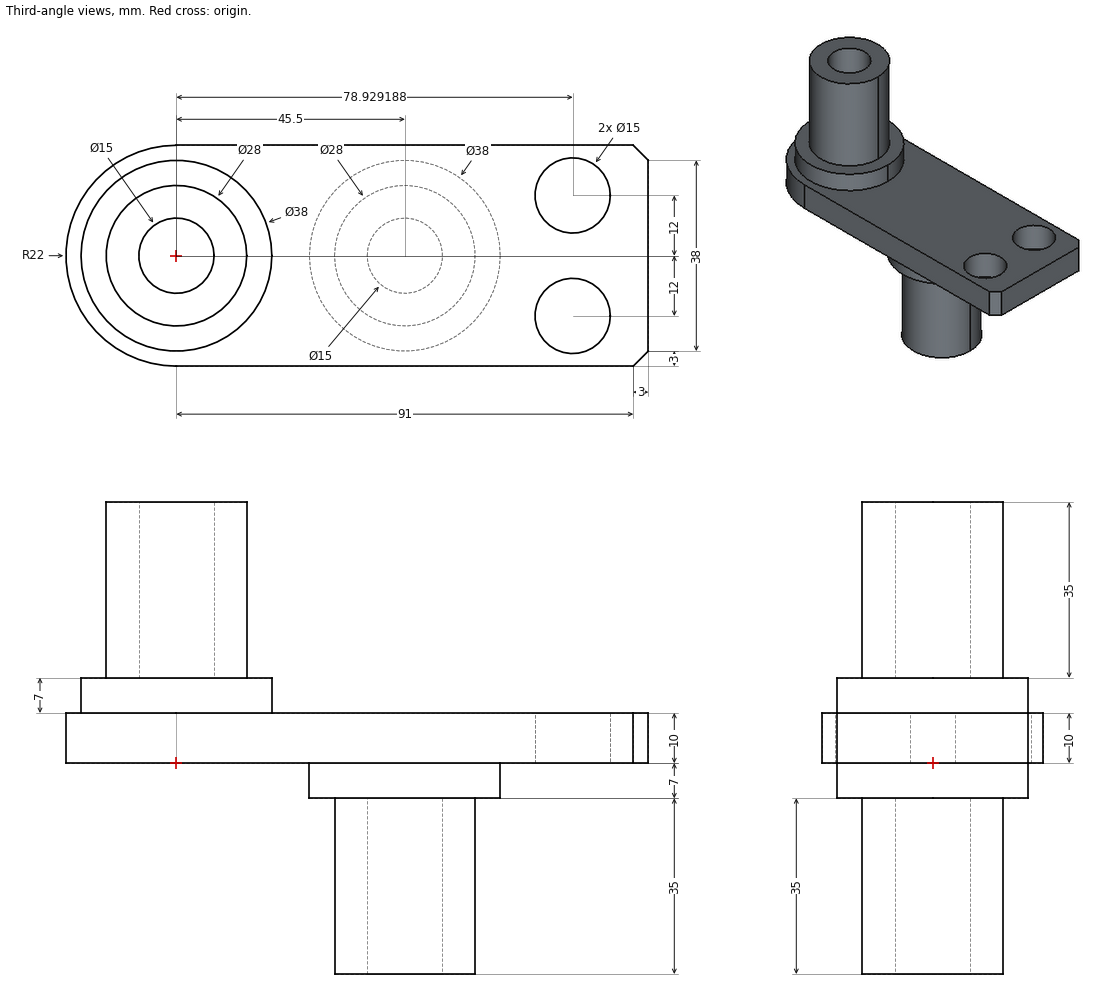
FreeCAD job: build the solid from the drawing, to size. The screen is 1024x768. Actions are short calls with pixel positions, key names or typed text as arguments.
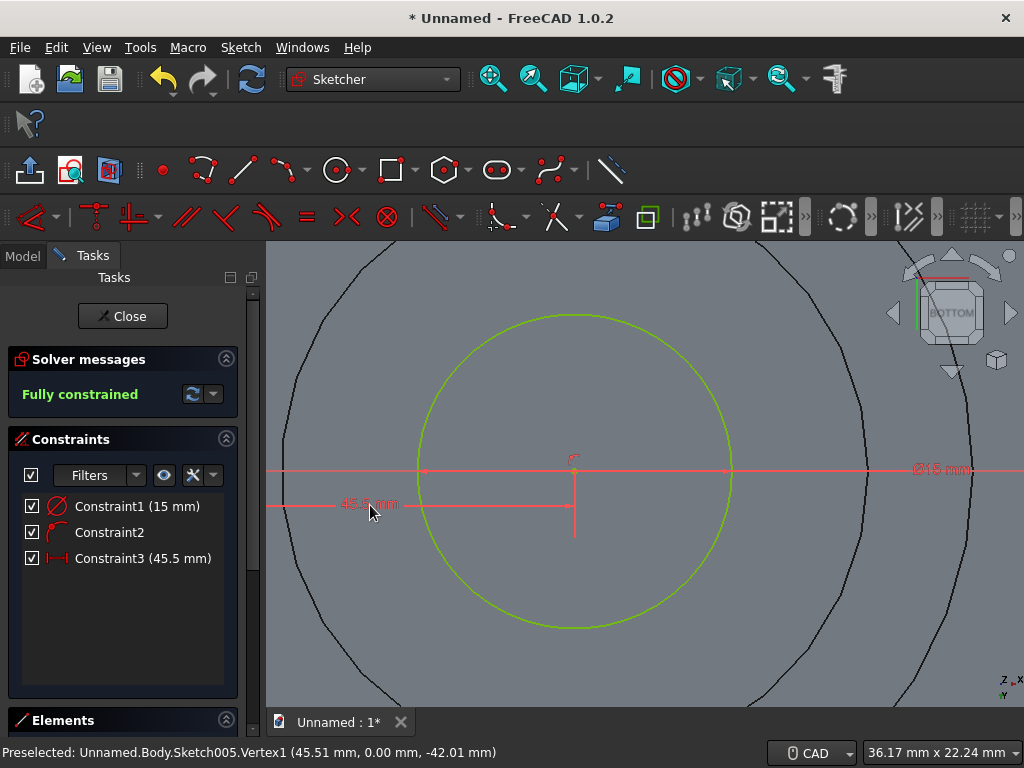
click(123, 316)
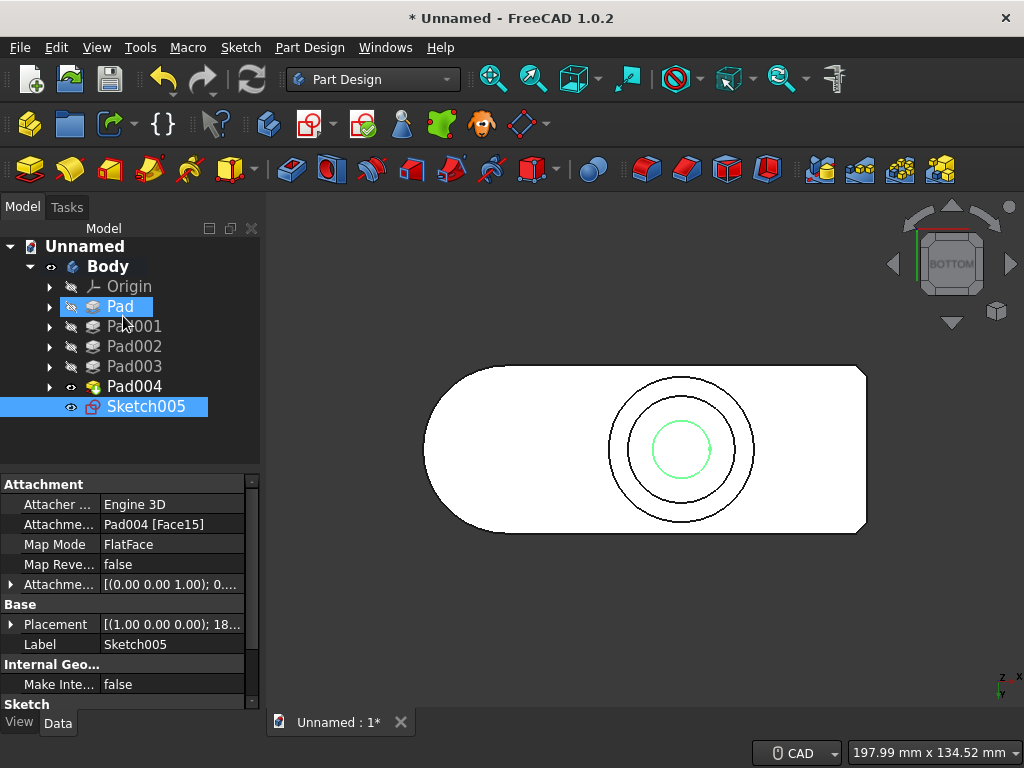
click(292, 170)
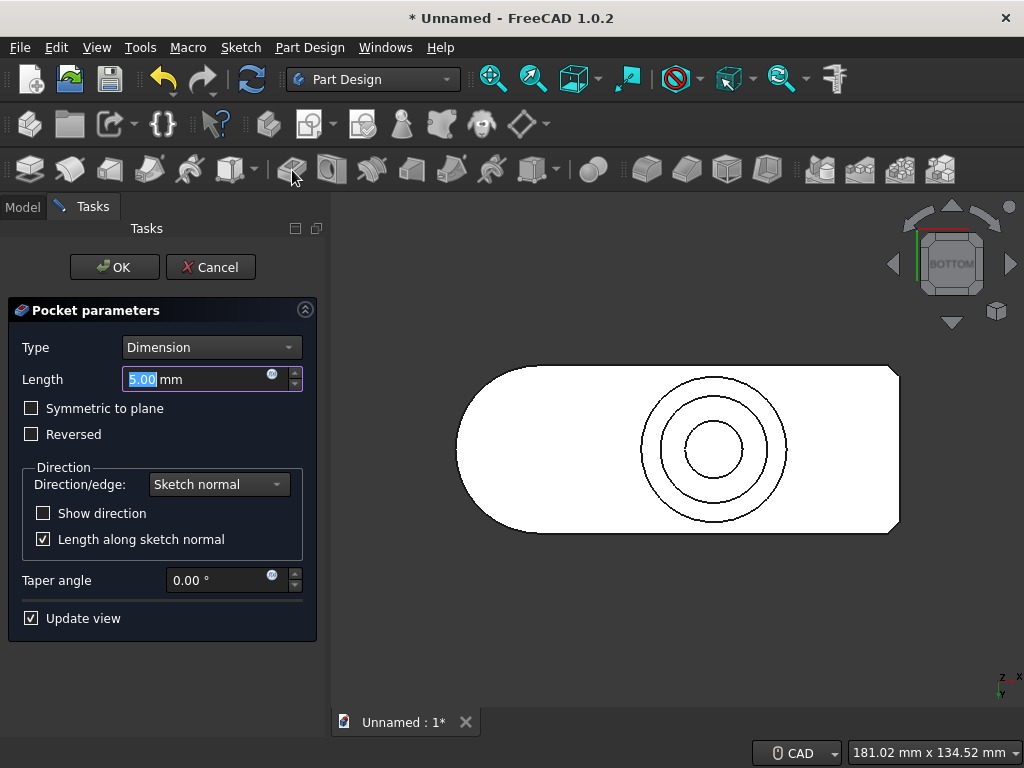
text(35)
key(Tab)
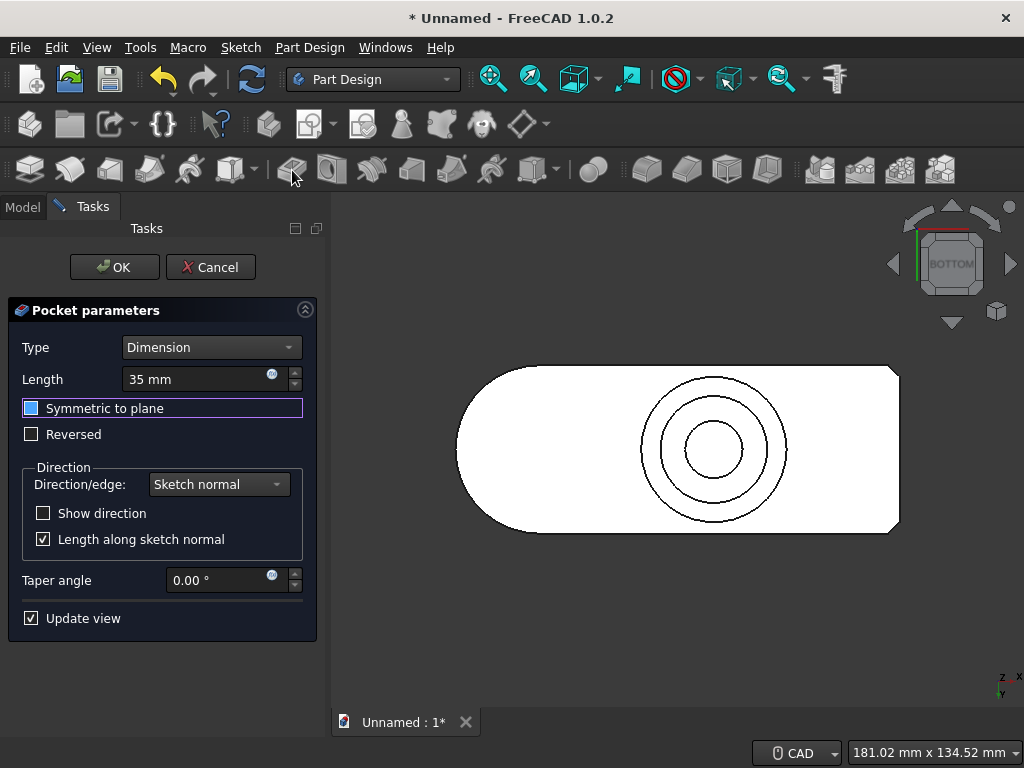
click(115, 267)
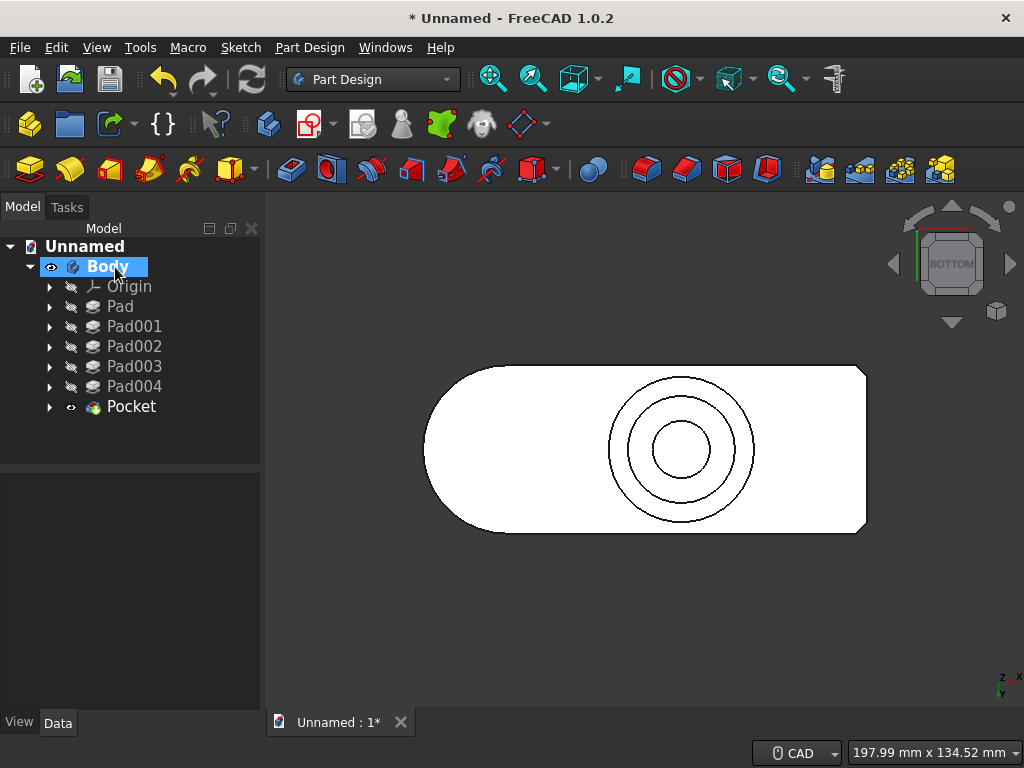
key(0)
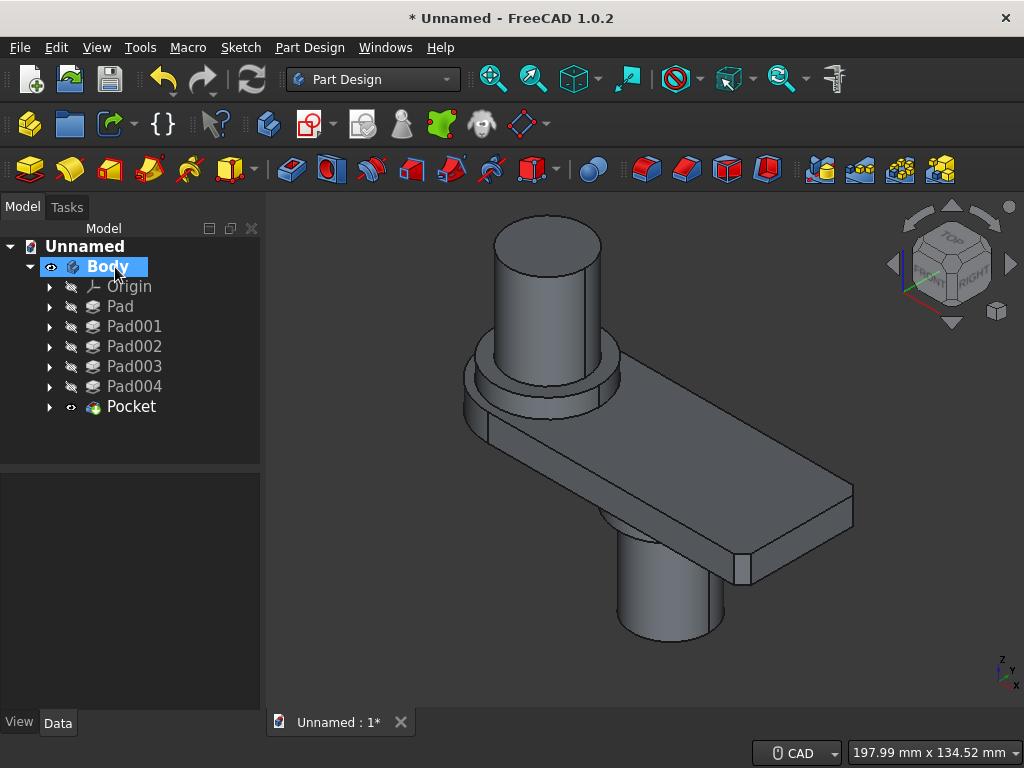
click(494, 80)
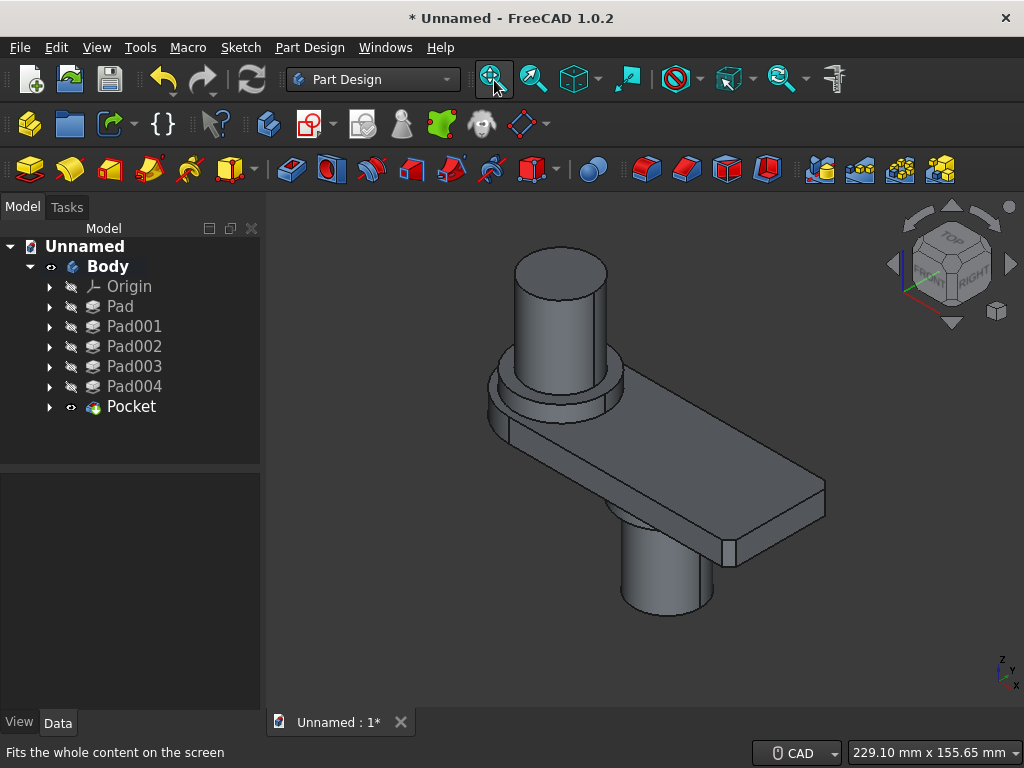
click(561, 273)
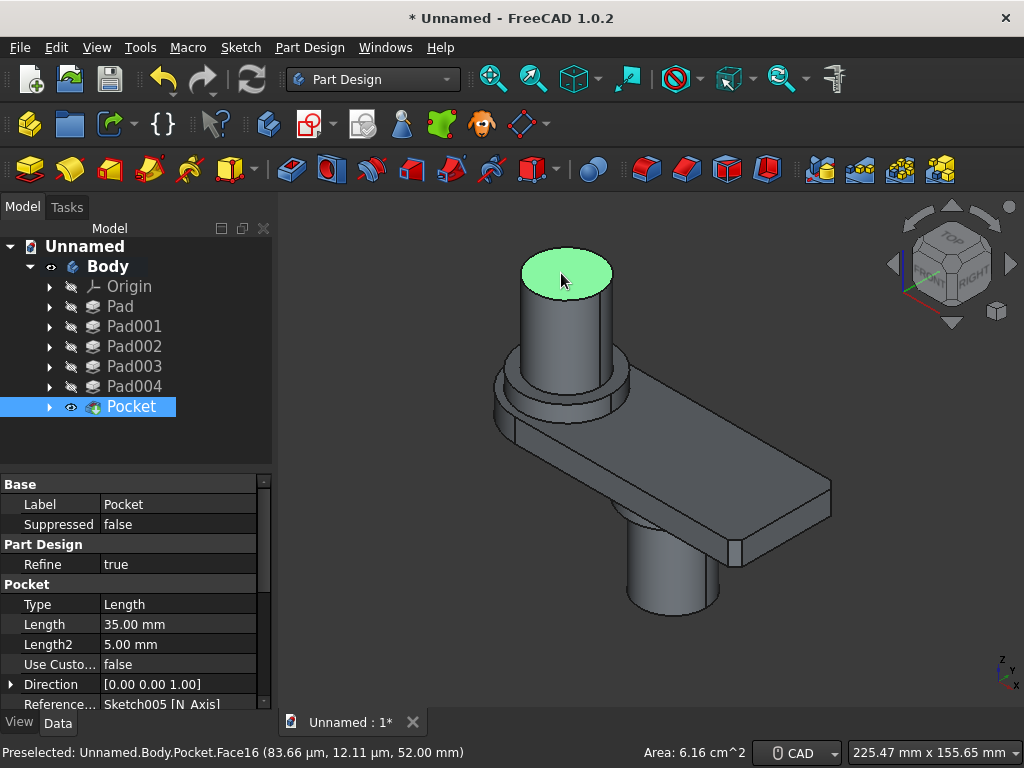
click(310, 124)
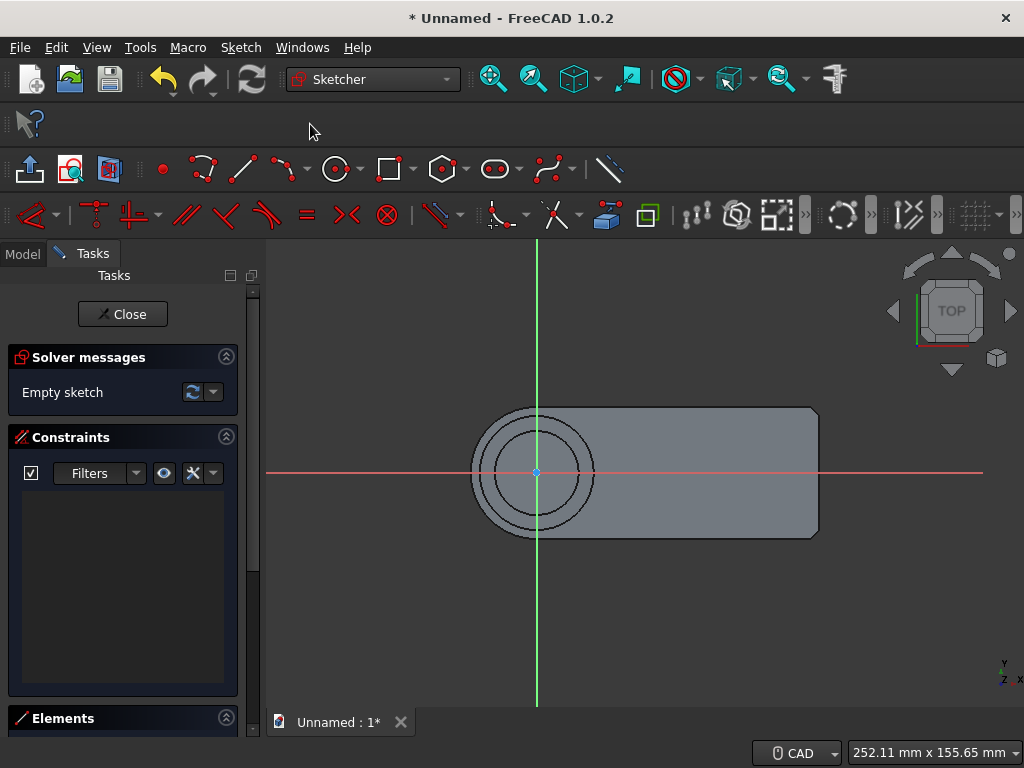
scroll(529, 473, up, 9)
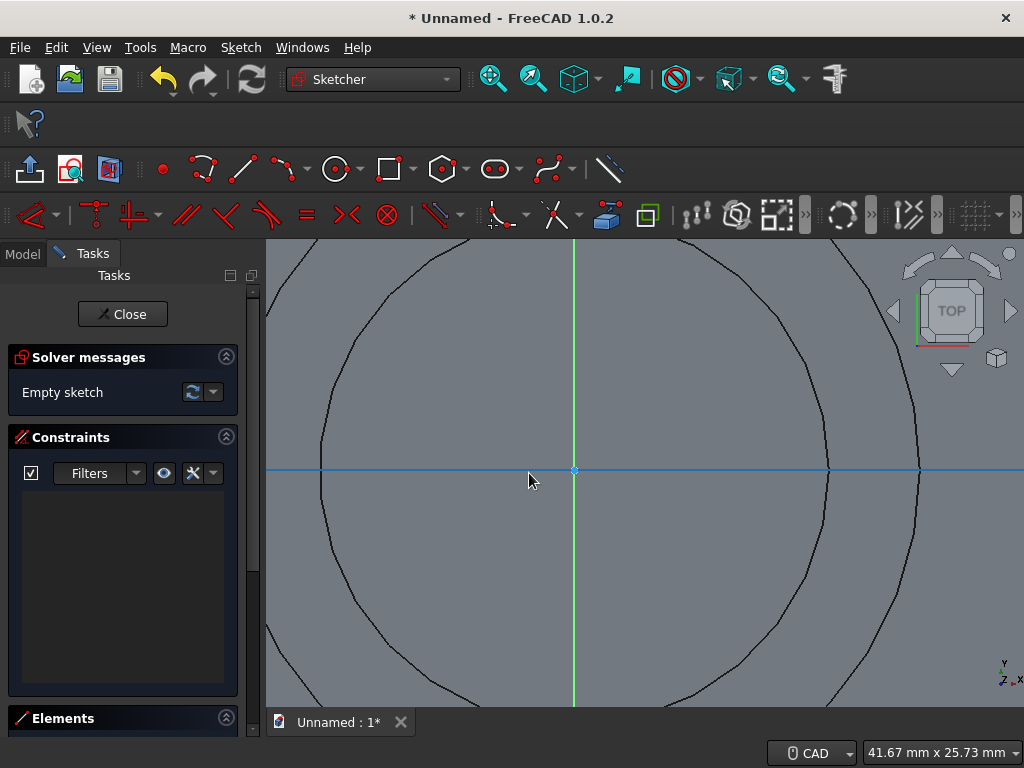
click(336, 170)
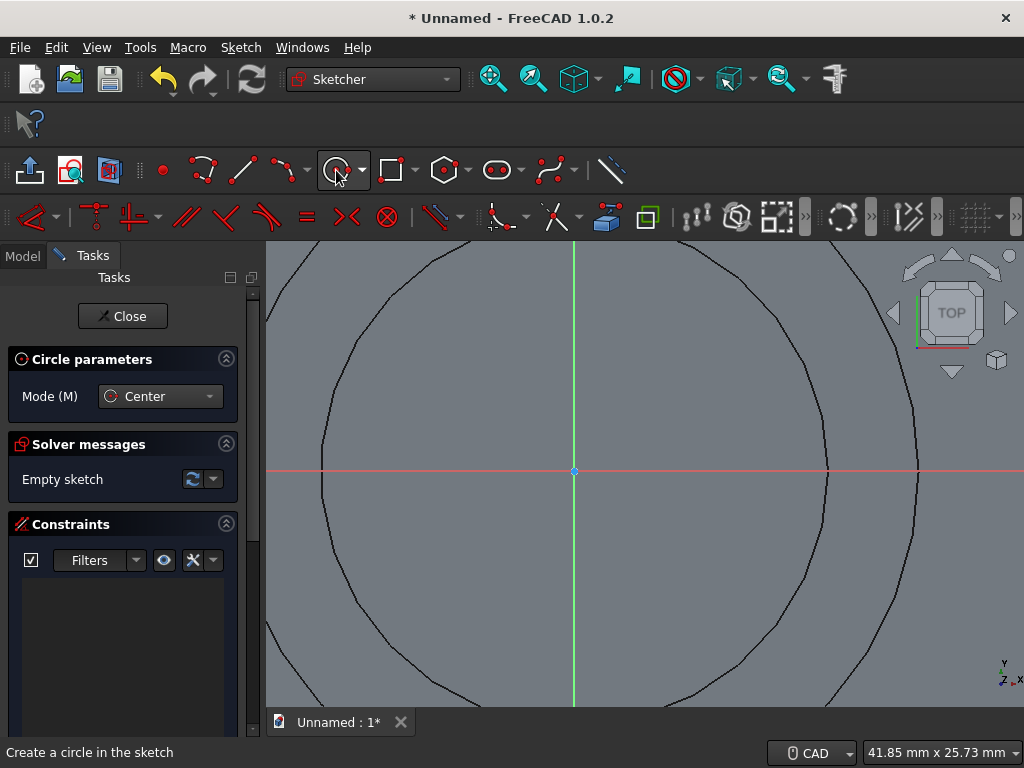
click(574, 471)
move(671, 375)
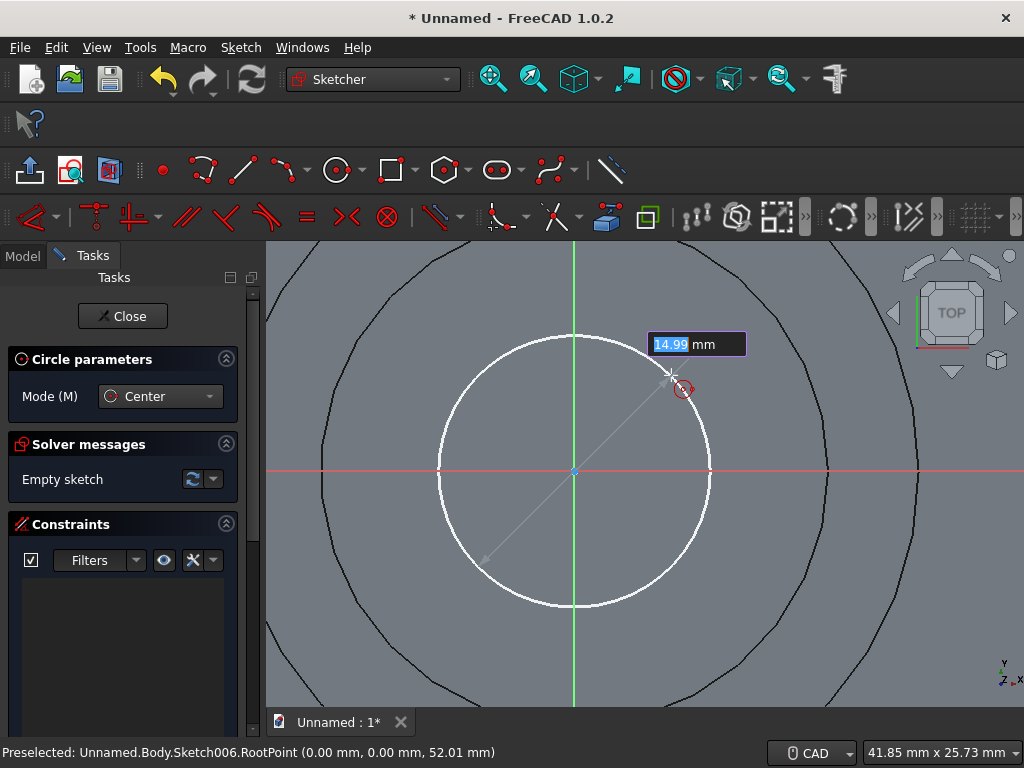
text(15)
key(Return)
key(Escape)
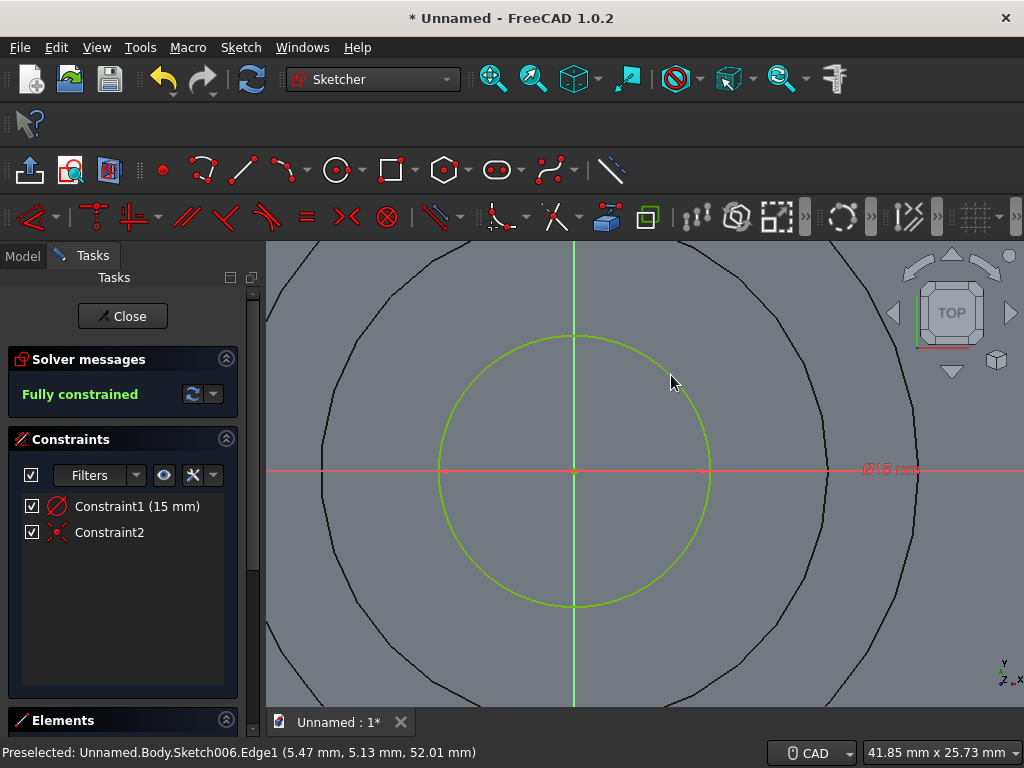
click(123, 316)